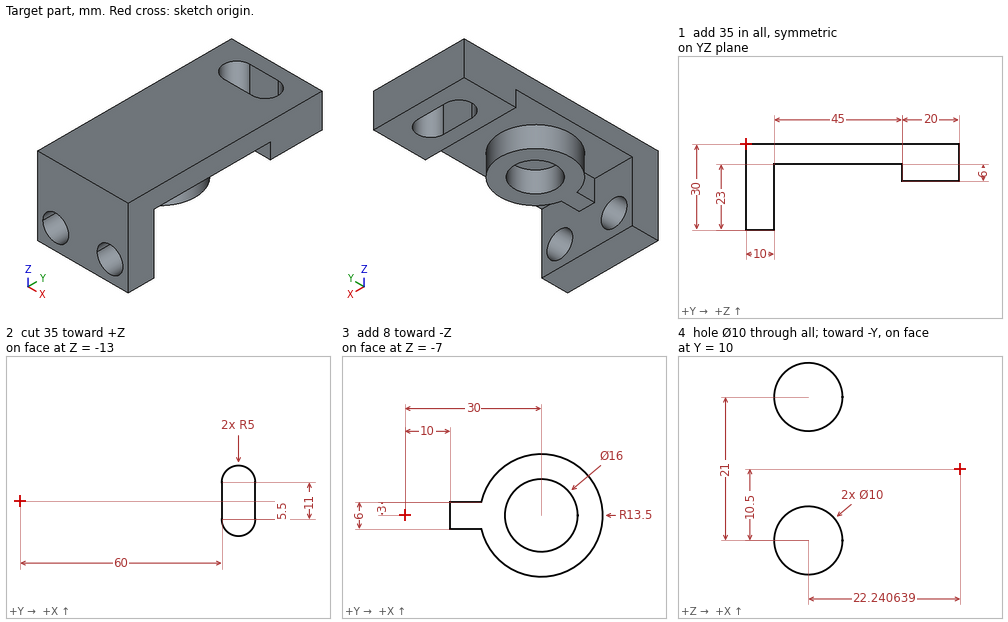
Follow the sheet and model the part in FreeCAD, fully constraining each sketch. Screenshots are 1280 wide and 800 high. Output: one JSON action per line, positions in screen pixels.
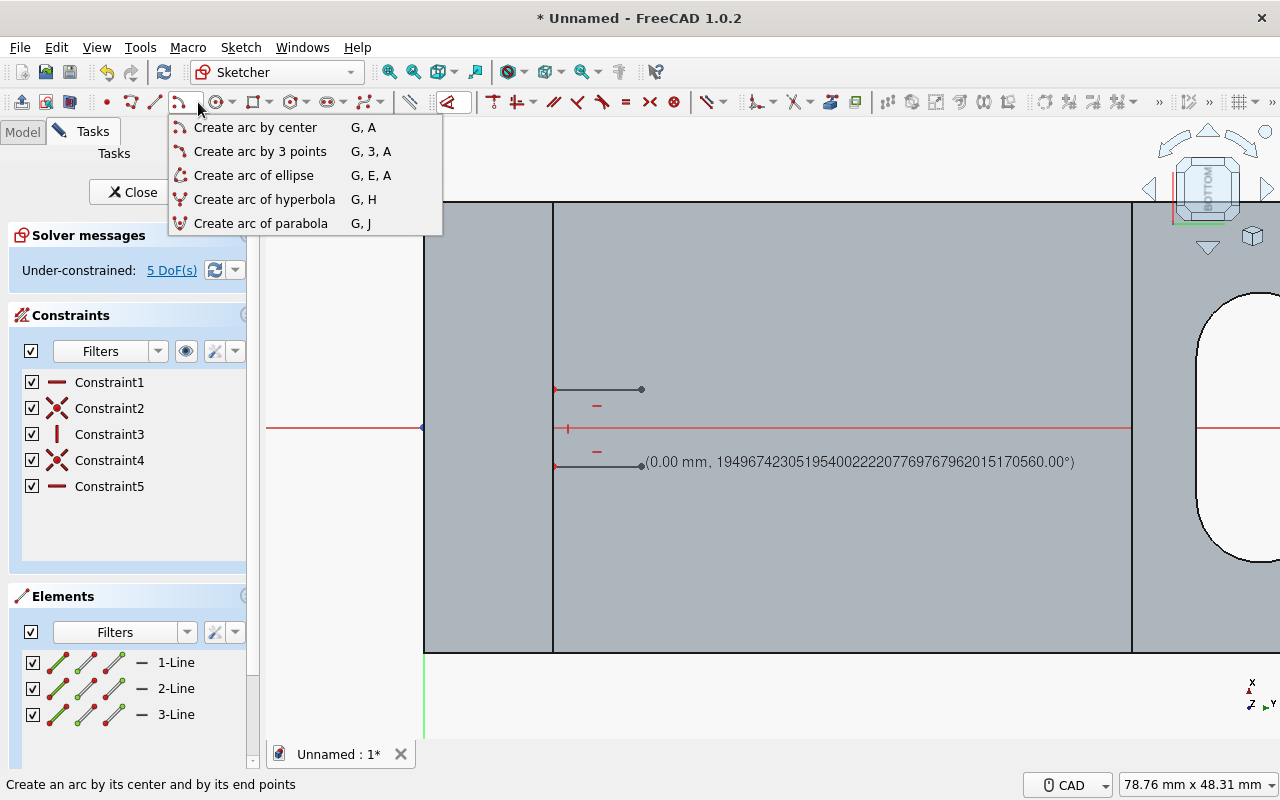
{"action": "left_click", "coordinate": [306, 151]}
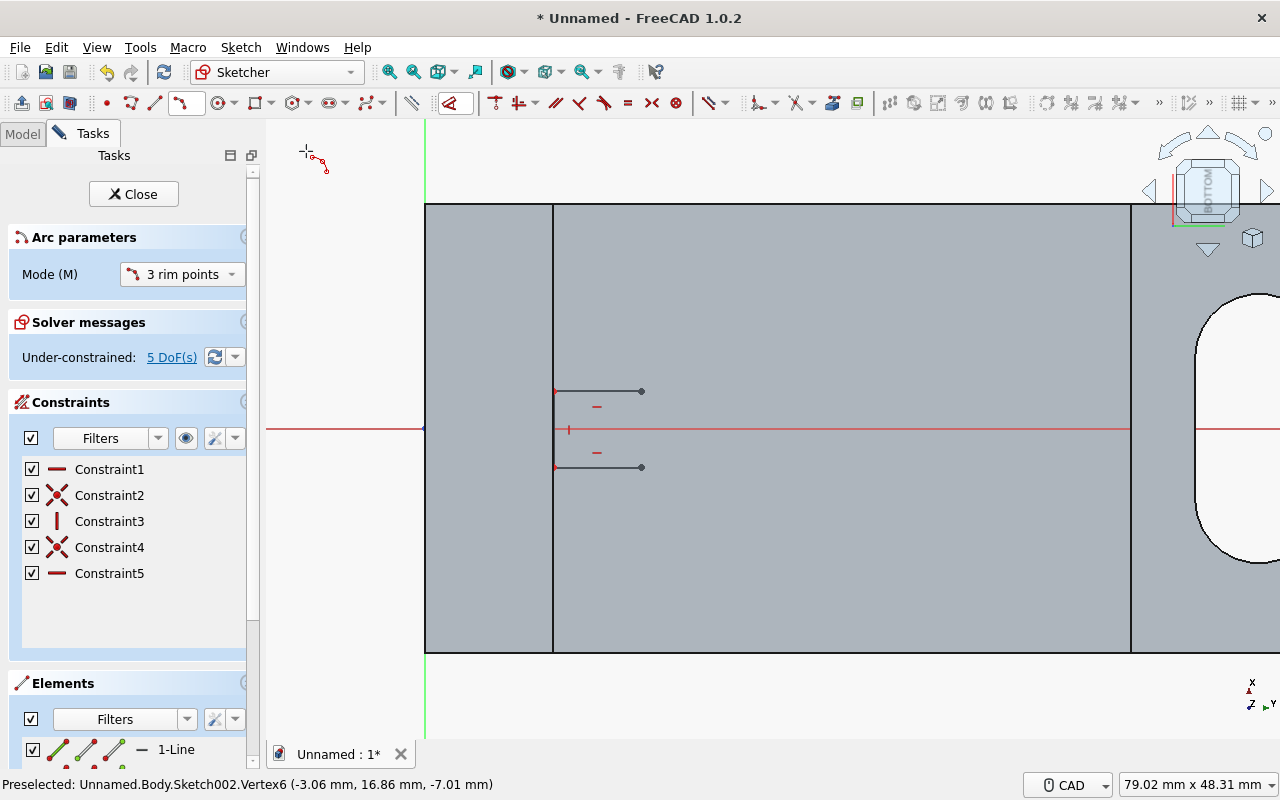
{"action": "left_click", "coordinate": [641, 468]}
{"action": "left_click", "coordinate": [641, 391]}
{"action": "left_click", "coordinate": [955, 524]}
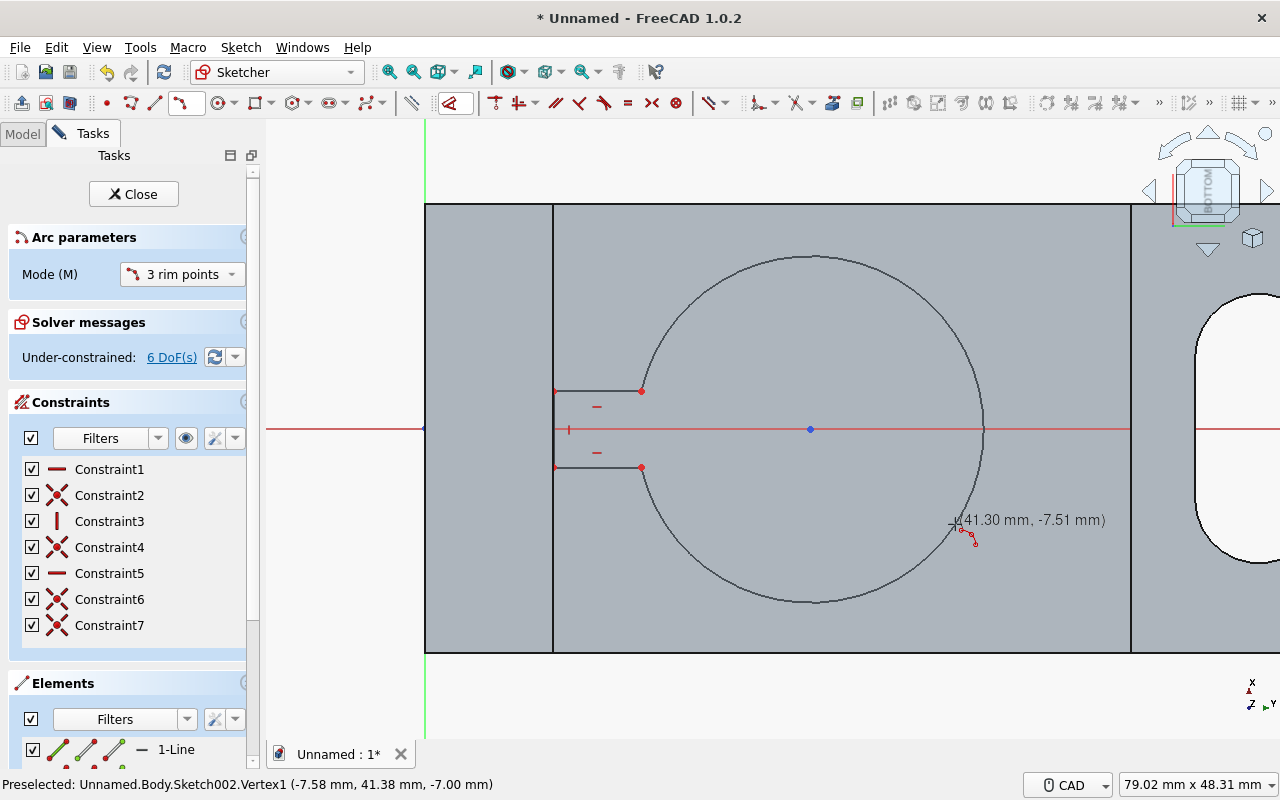
{"action": "left_click", "coordinate": [218, 104]}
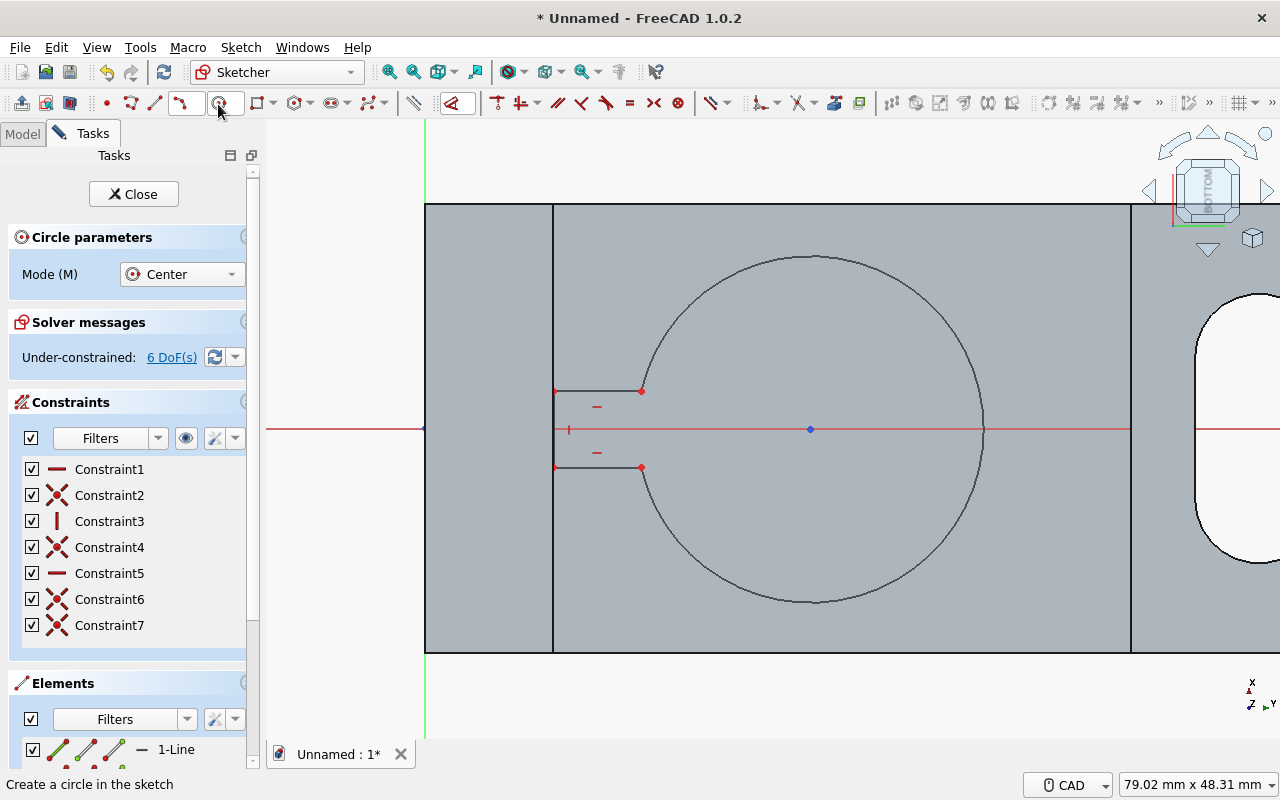
{"action": "left_click", "coordinate": [810, 429]}
{"action": "mouse_move", "coordinate": [883, 356]}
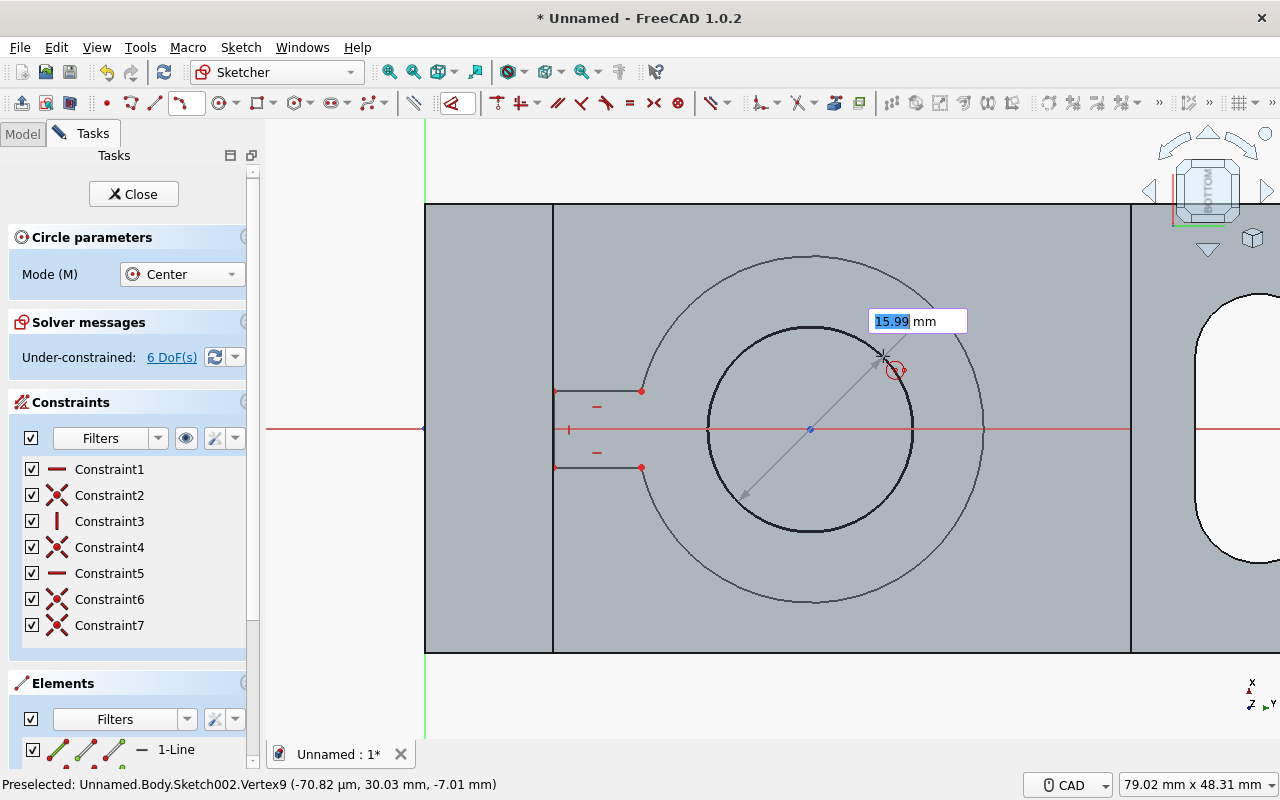
{"action": "type", "text": "16"}
{"action": "key", "text": "Return"}
{"action": "key", "text": "Escape"}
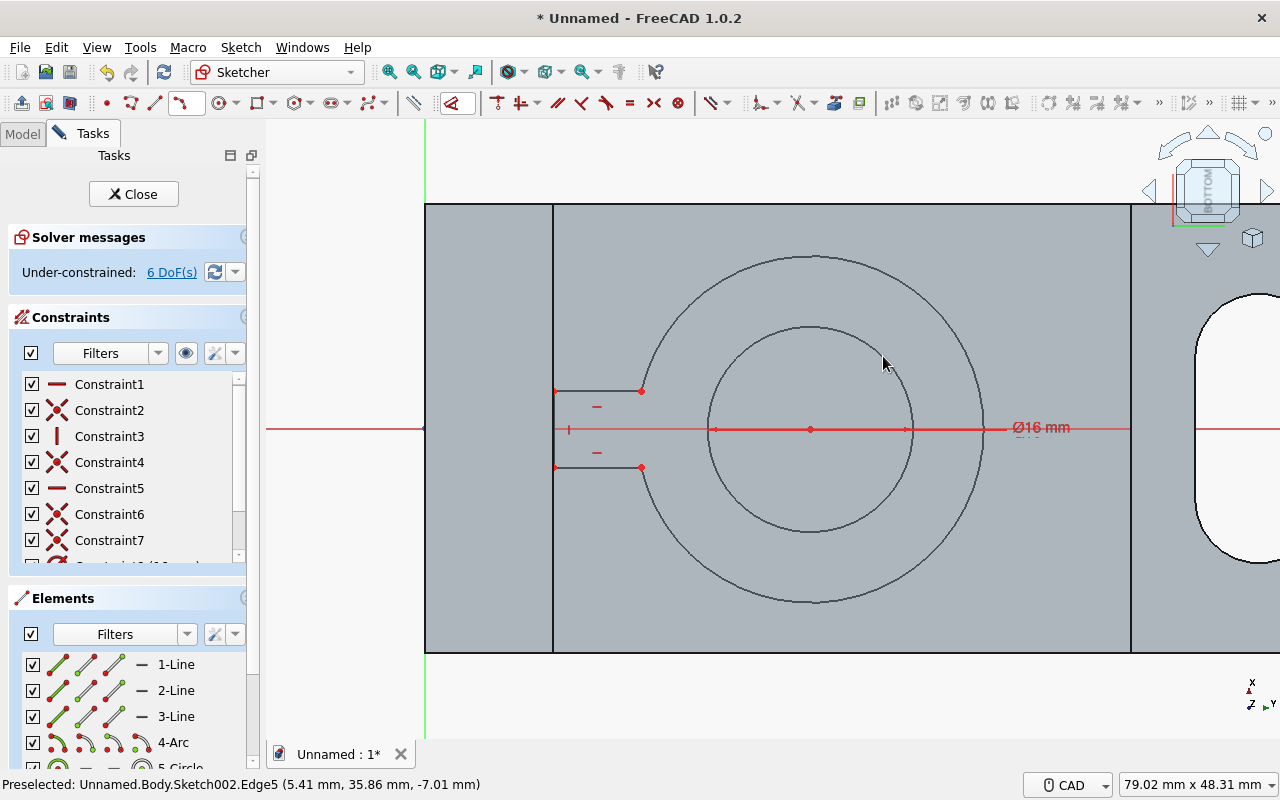
{"action": "left_click", "coordinate": [810, 429]}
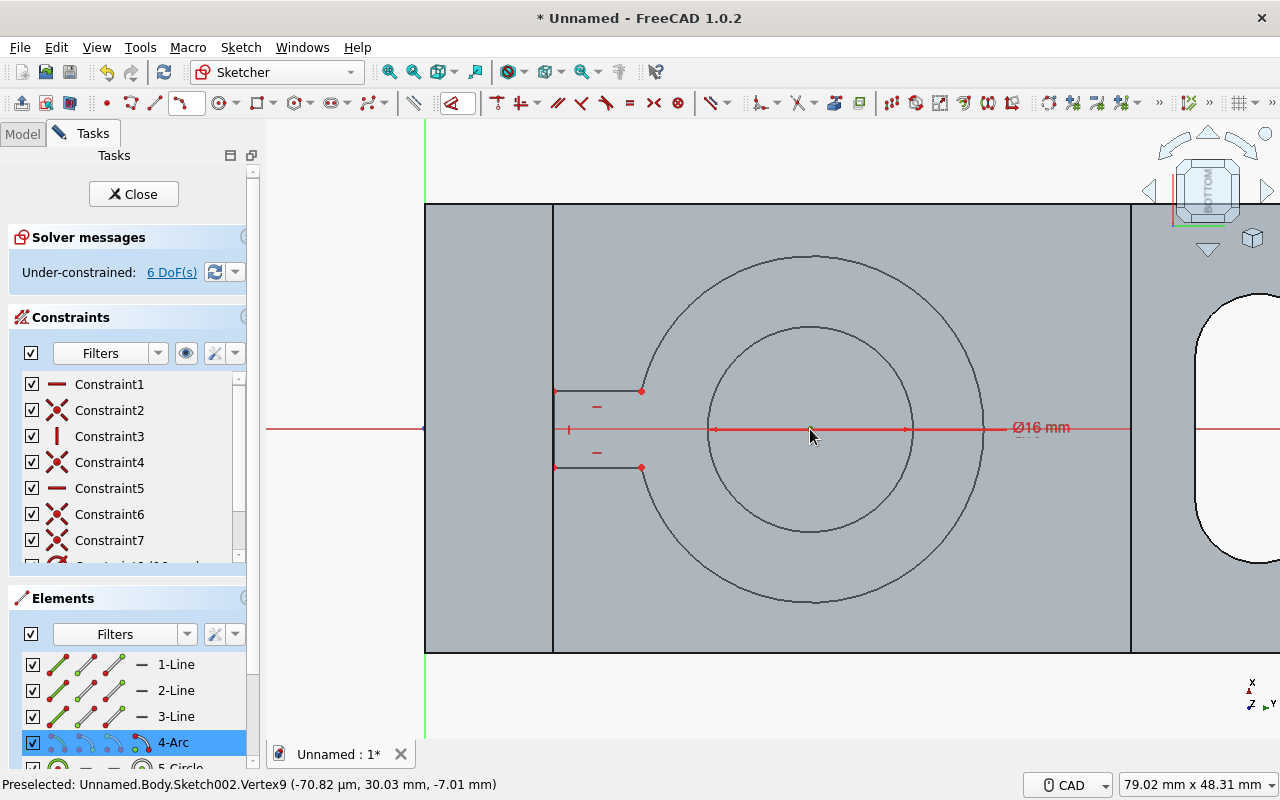
{"action": "left_click", "coordinate": [353, 429]}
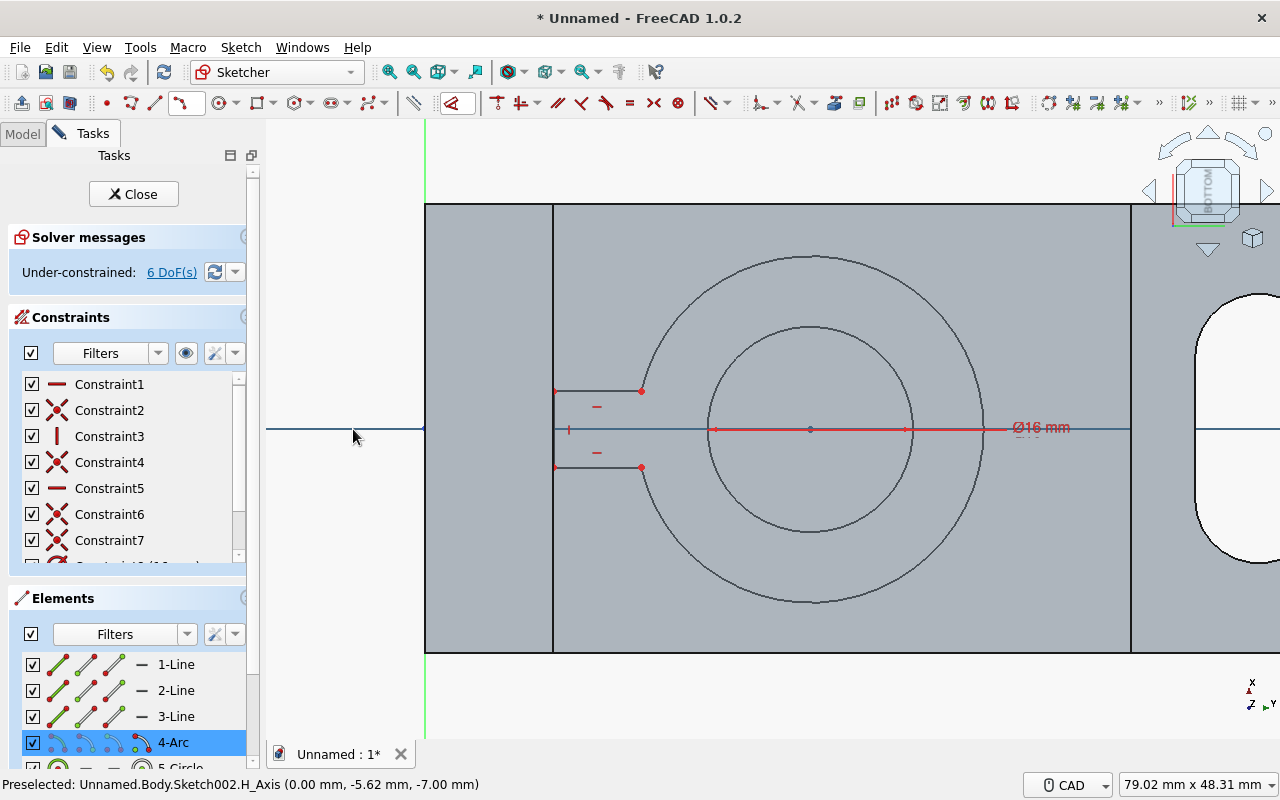
{"action": "left_click", "coordinate": [498, 104]}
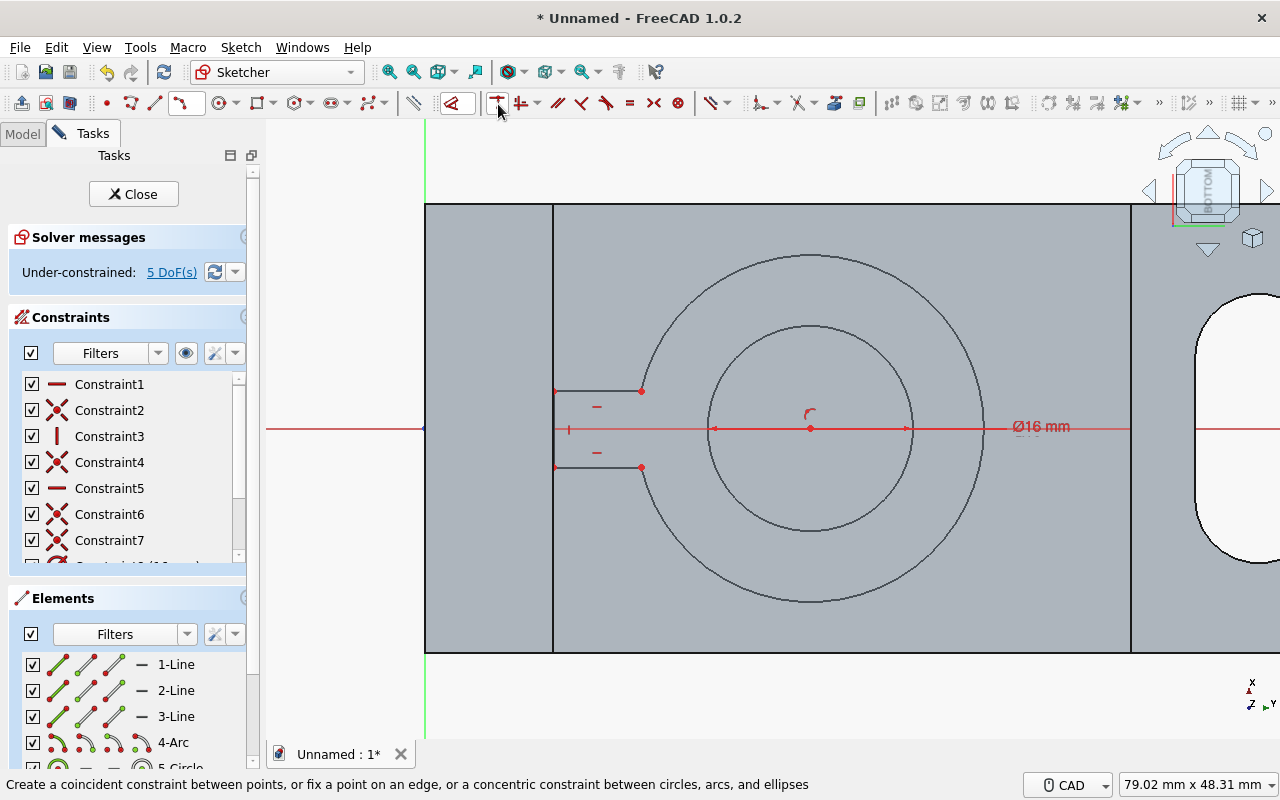
{"action": "left_click", "coordinate": [879, 588]}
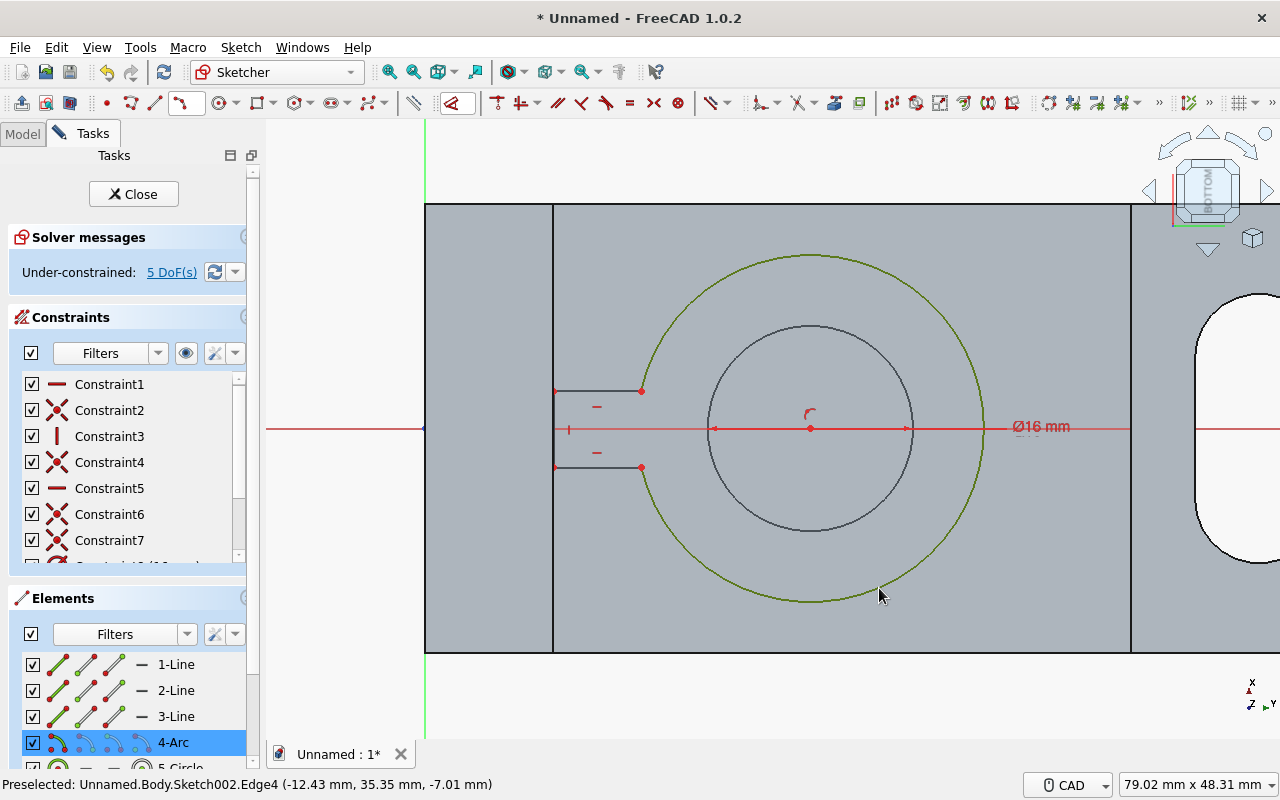
{"action": "key", "text": "k r"}